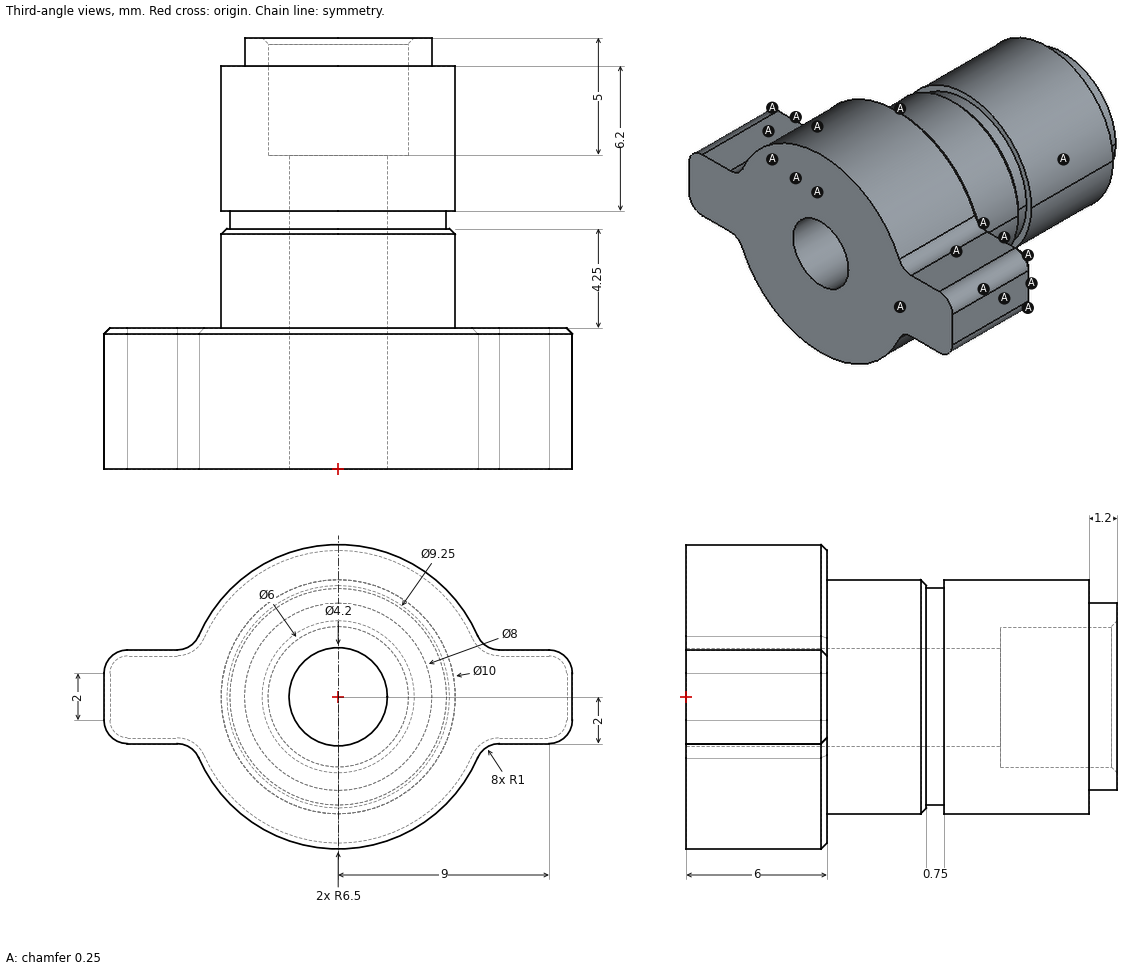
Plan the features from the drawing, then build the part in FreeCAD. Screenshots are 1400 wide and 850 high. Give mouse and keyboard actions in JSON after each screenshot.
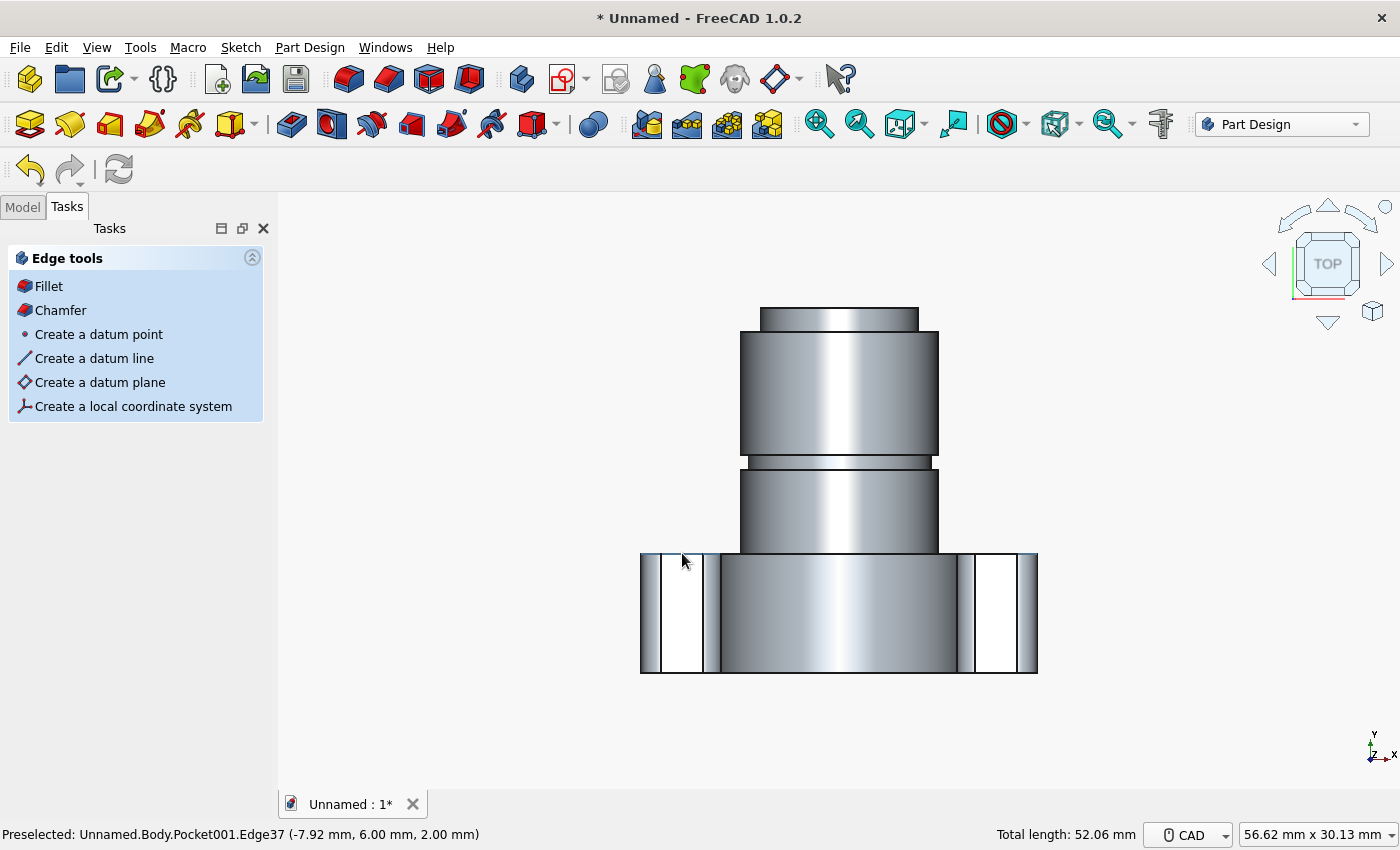
{"action": "left_click", "coordinate": [839, 553], "text": "ctrl"}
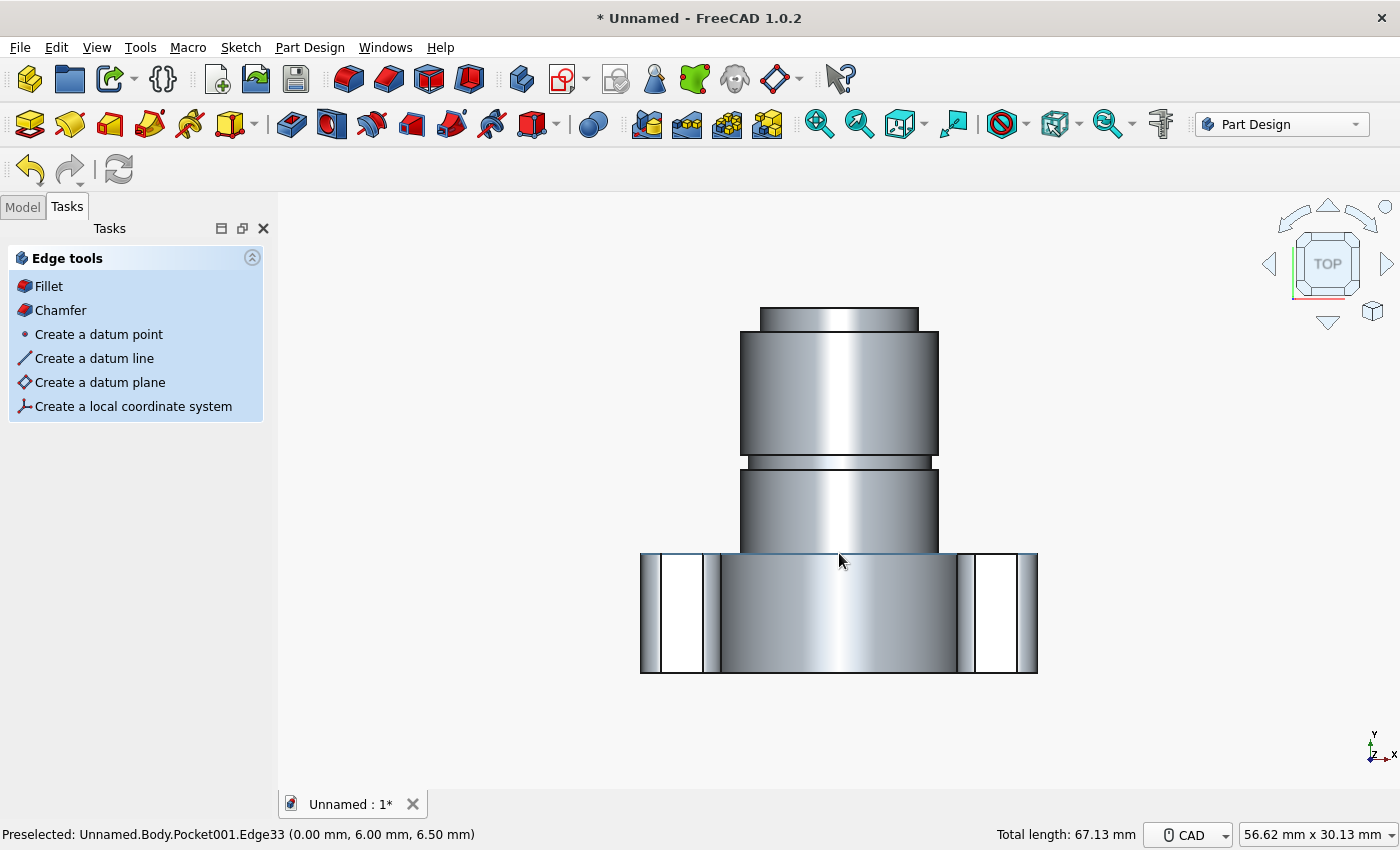
{"action": "left_click", "coordinate": [964, 553], "text": "ctrl"}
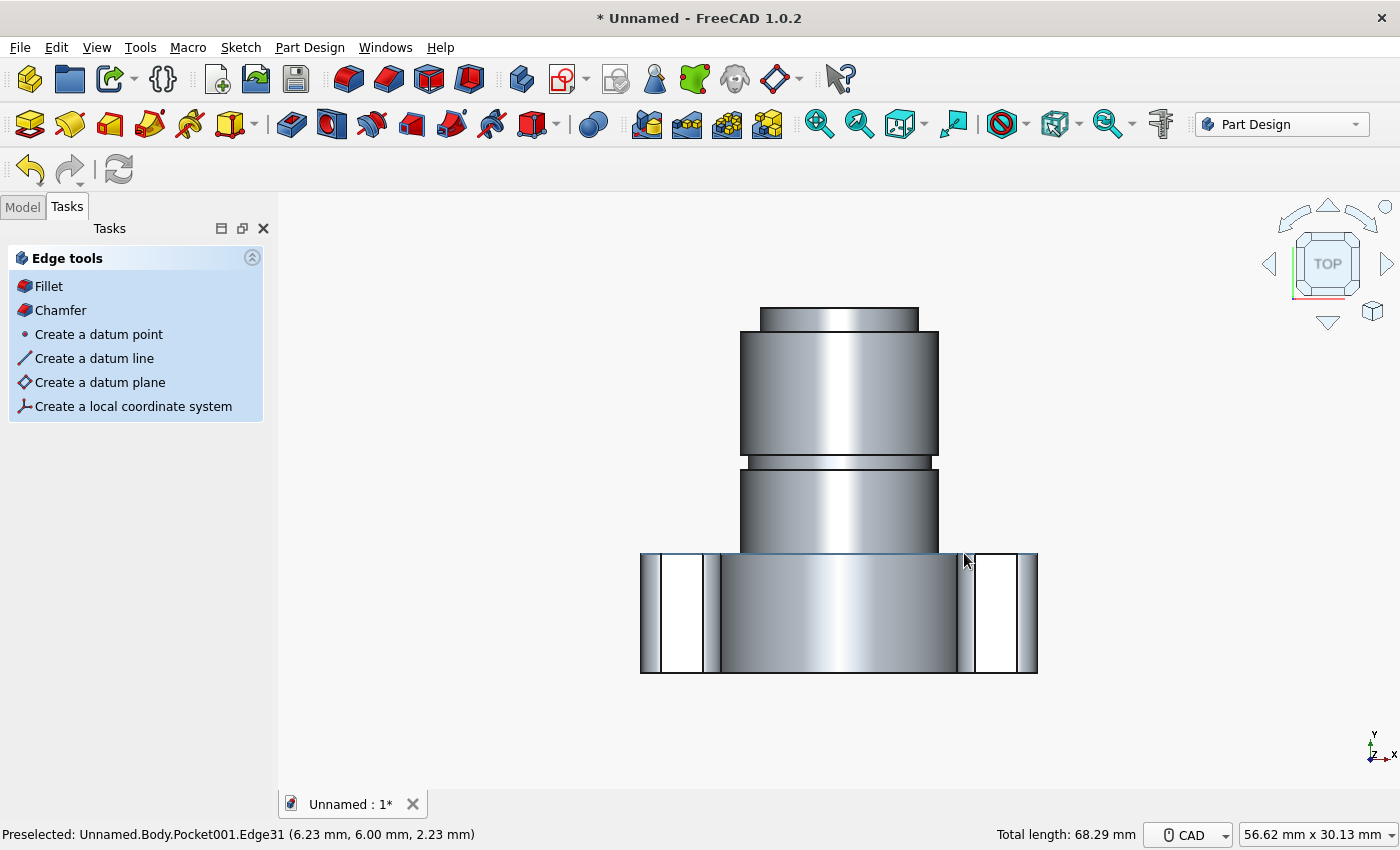
{"action": "left_click", "coordinate": [759, 469], "text": "ctrl"}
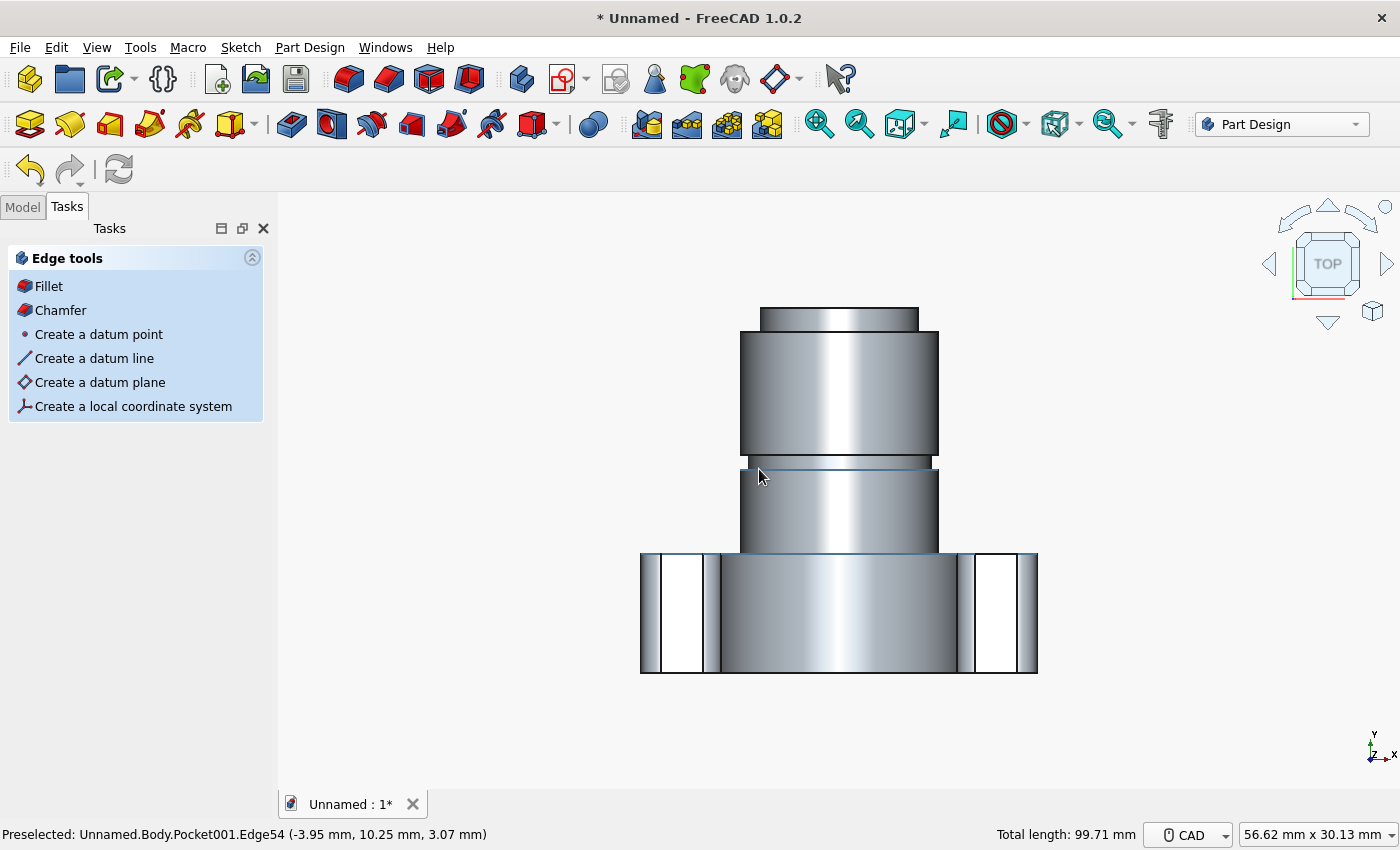
{"action": "left_click", "coordinate": [996, 553], "text": "ctrl"}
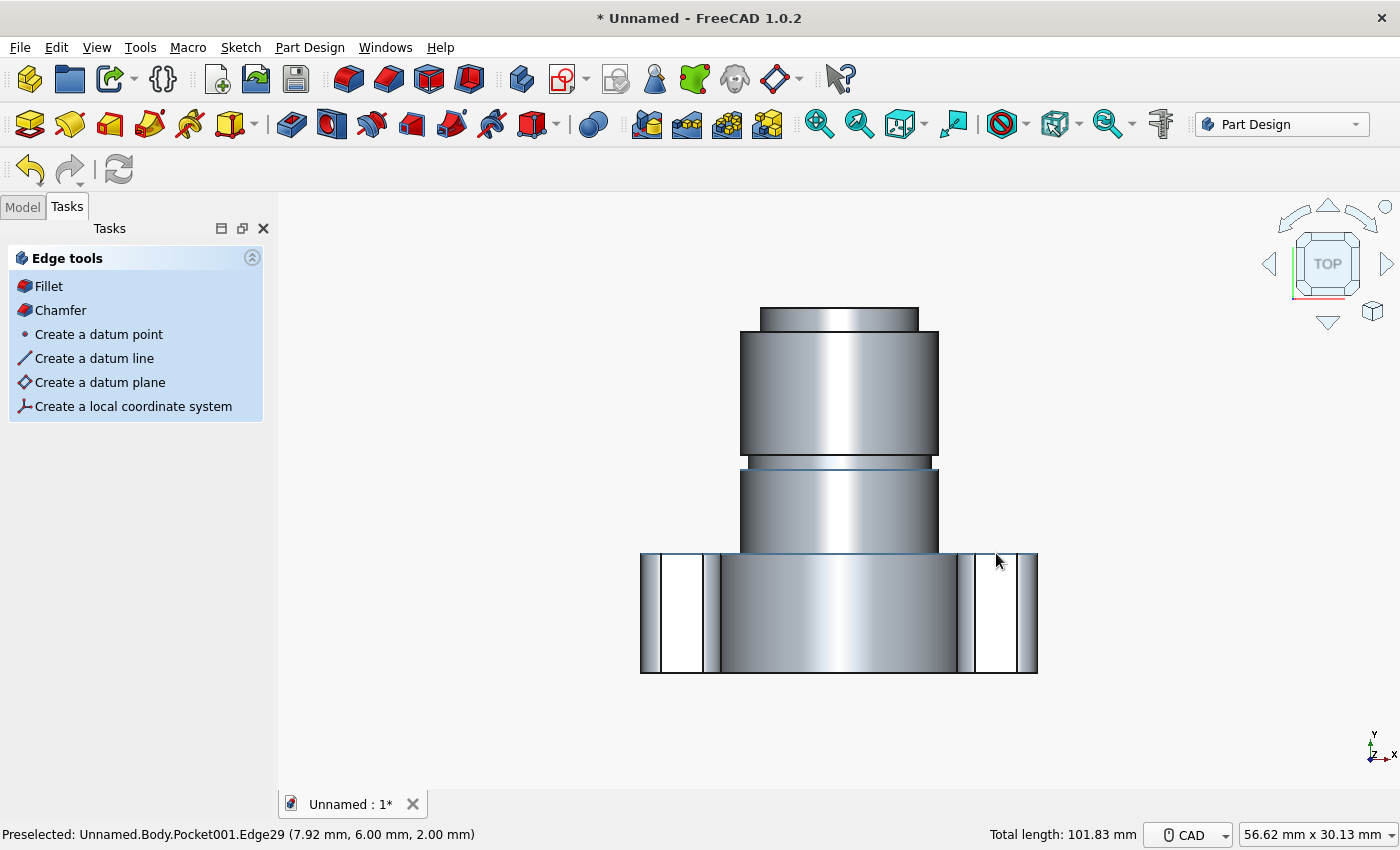
{"action": "key", "text": "1"}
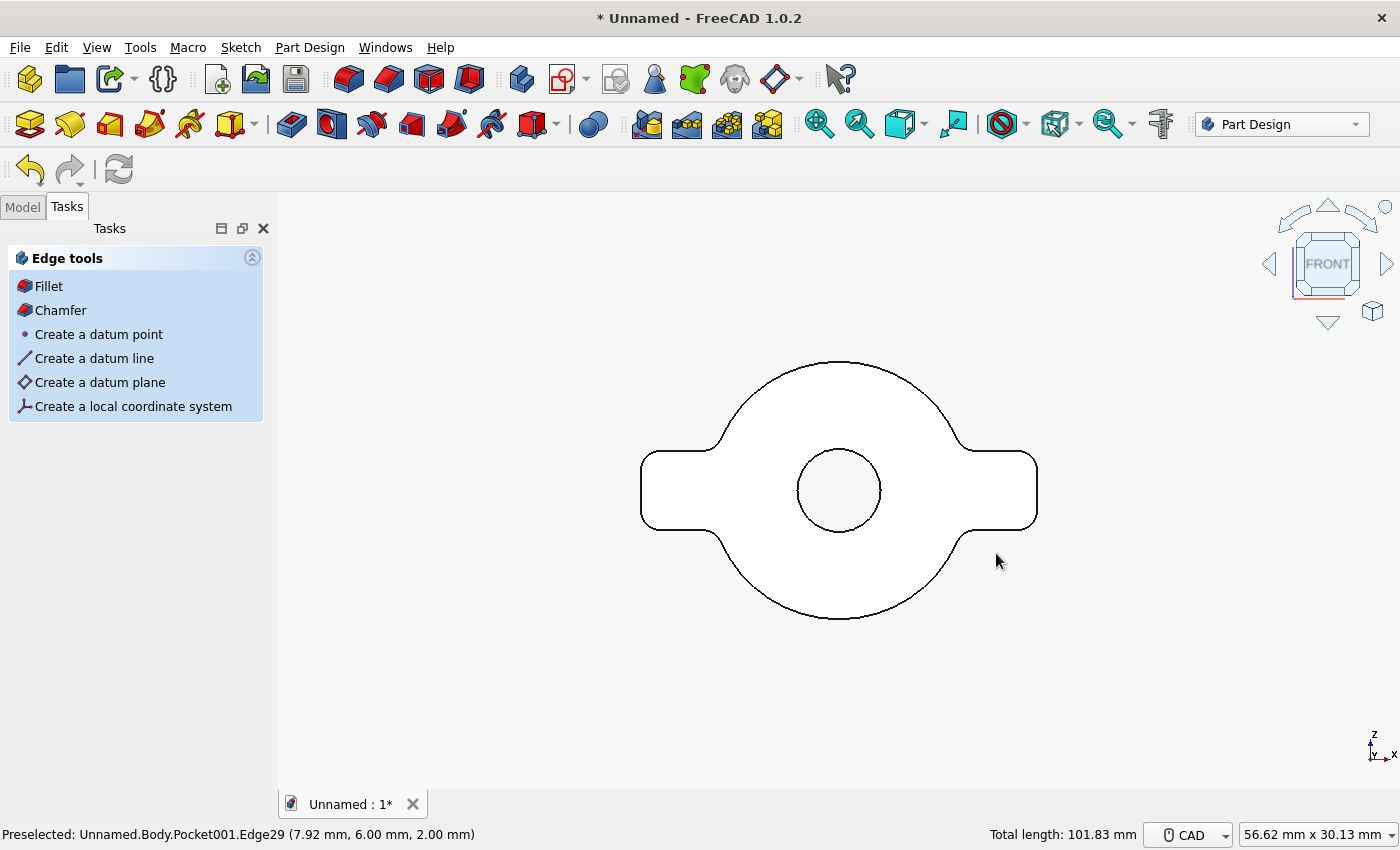
{"action": "left_click", "coordinate": [820, 124]}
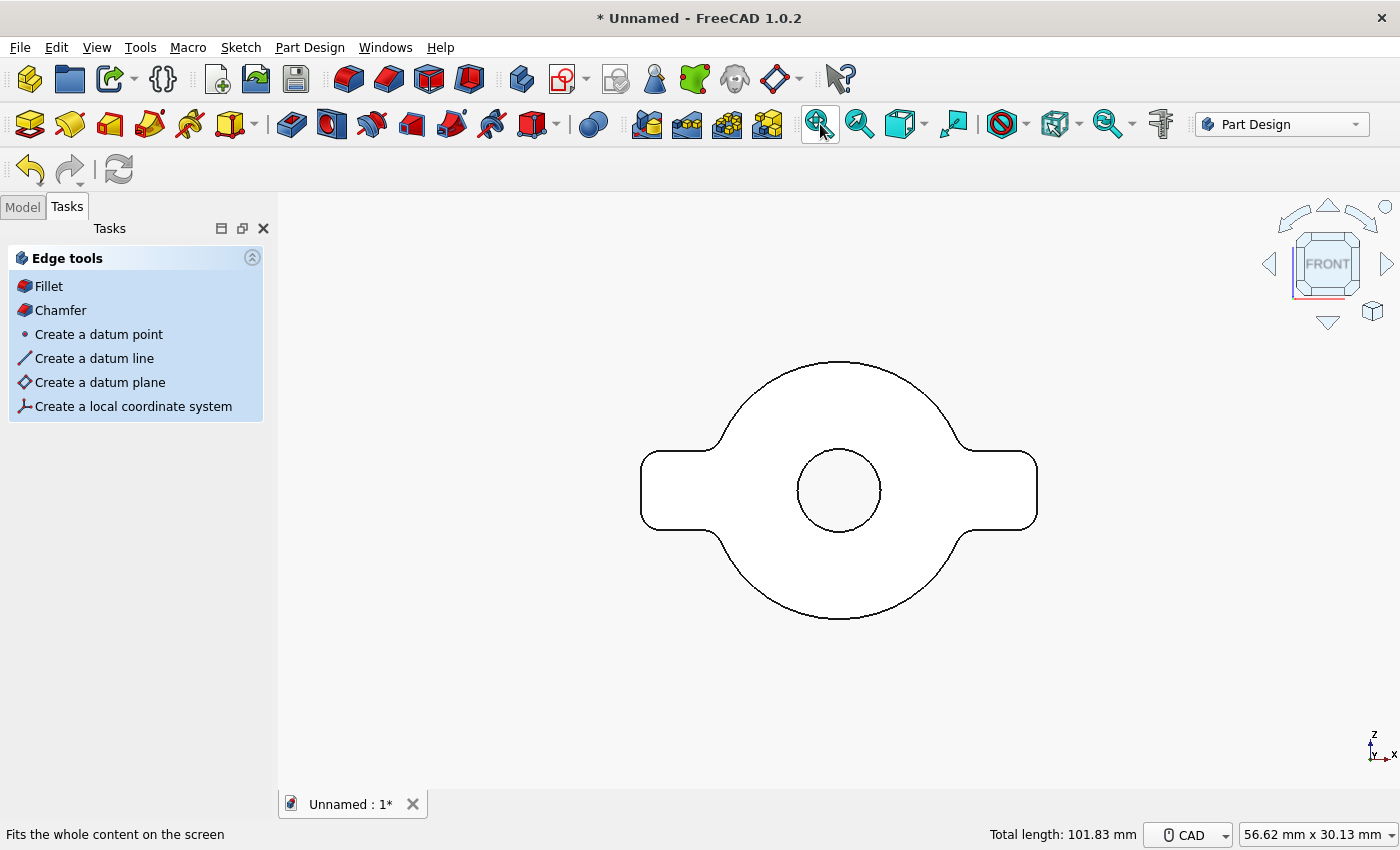
{"action": "key", "text": "3"}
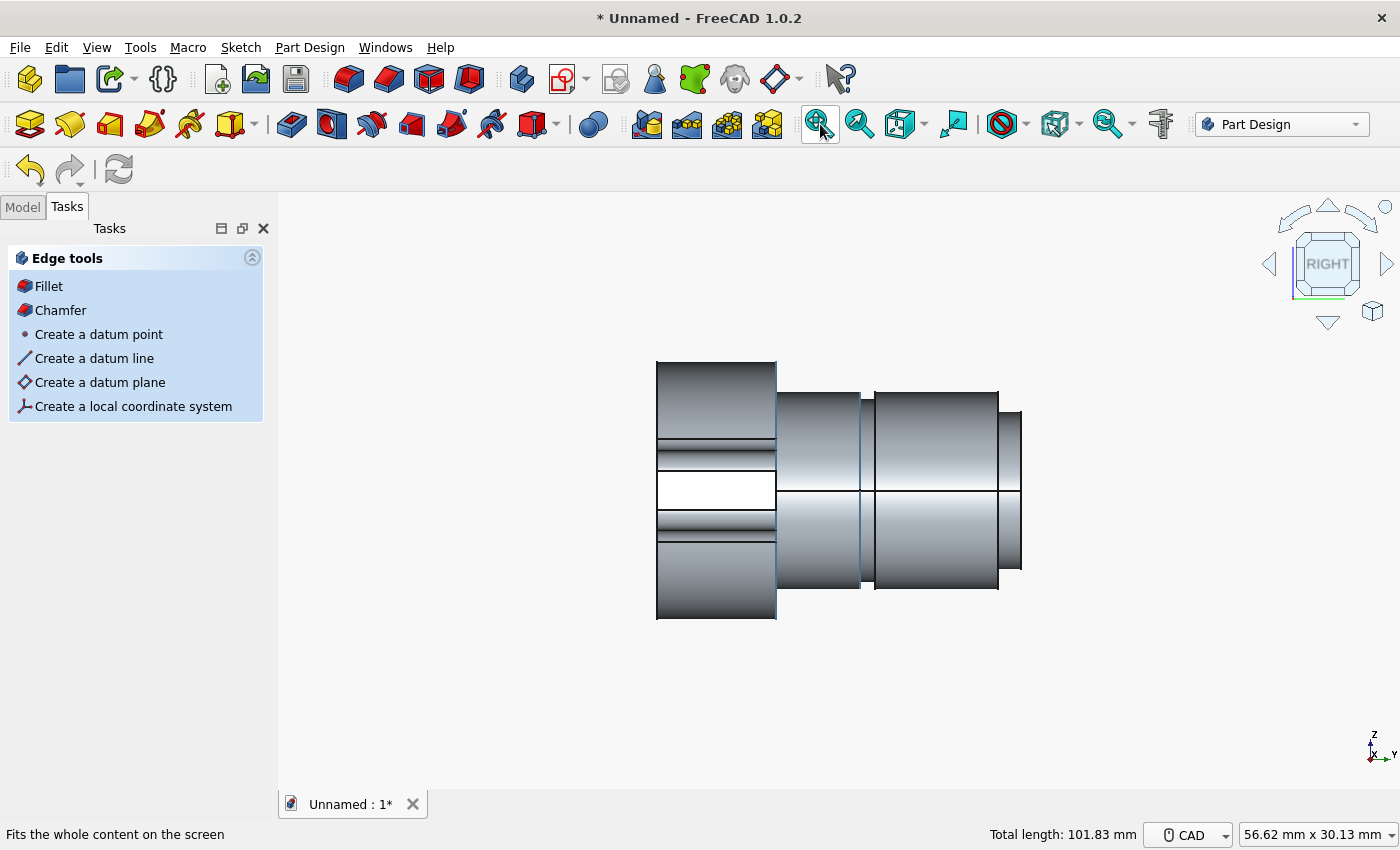
{"action": "left_click", "coordinate": [820, 124]}